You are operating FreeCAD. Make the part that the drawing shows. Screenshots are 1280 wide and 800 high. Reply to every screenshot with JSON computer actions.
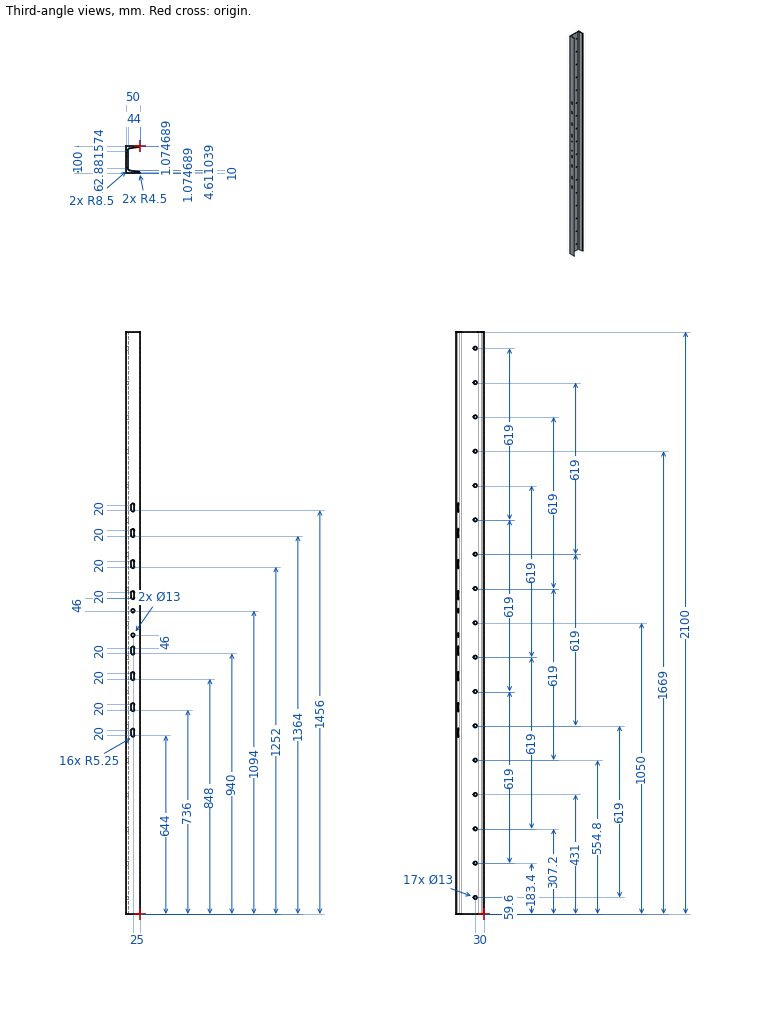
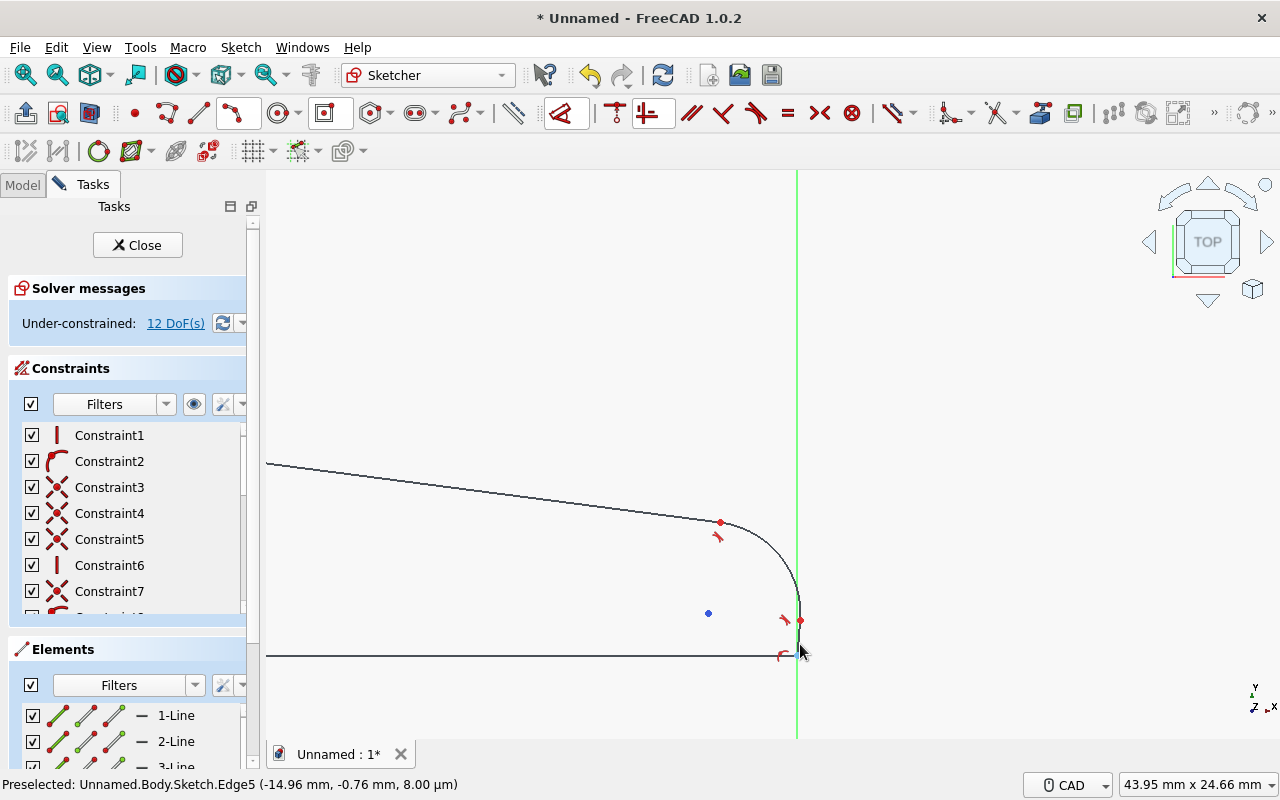
{"action": "left_click", "coordinate": [799, 642]}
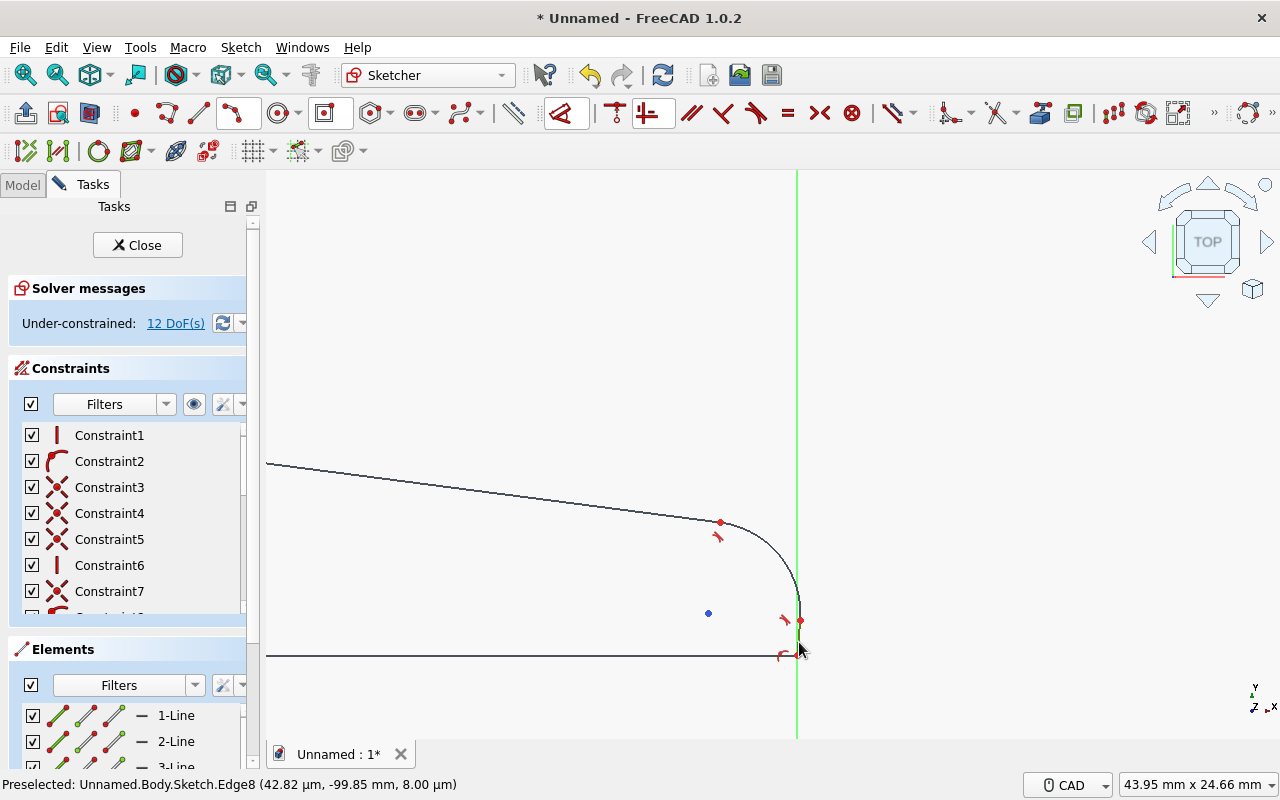
{"action": "left_click", "coordinate": [670, 114]}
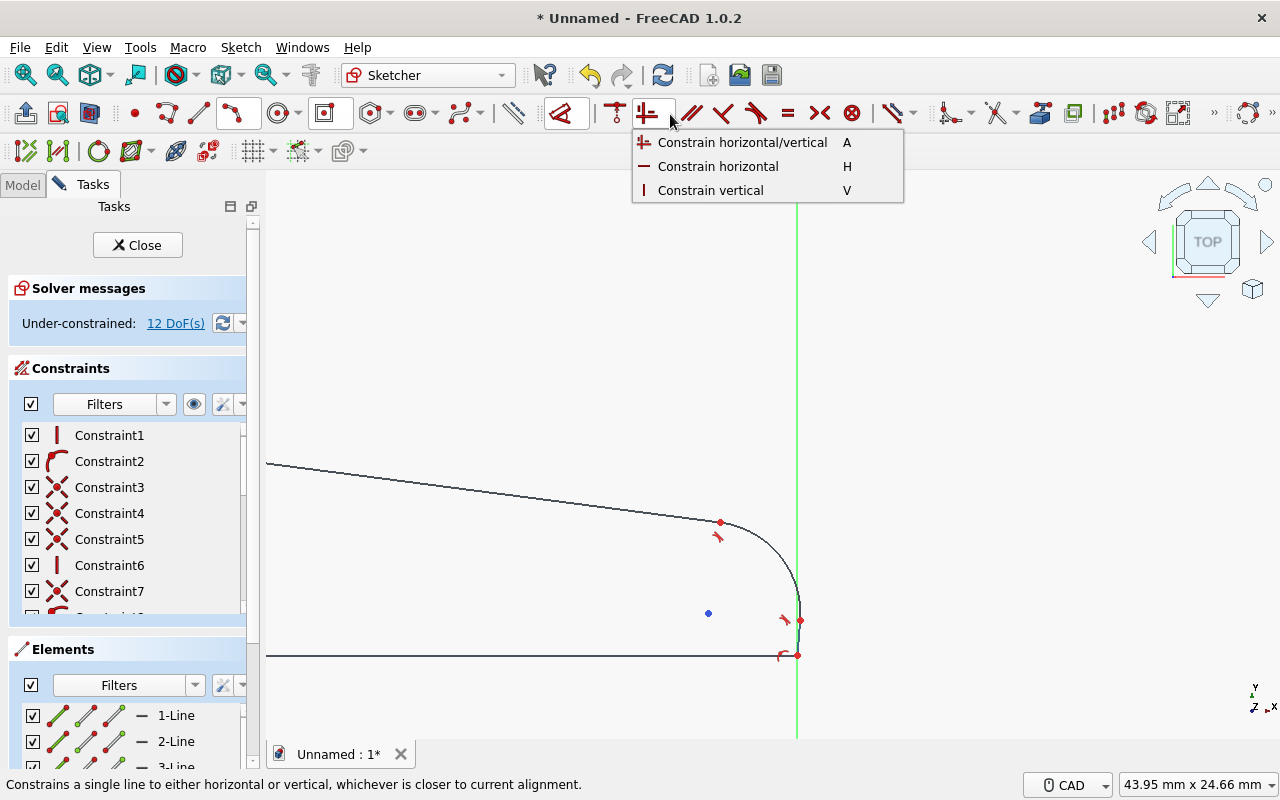
{"action": "left_click", "coordinate": [768, 190]}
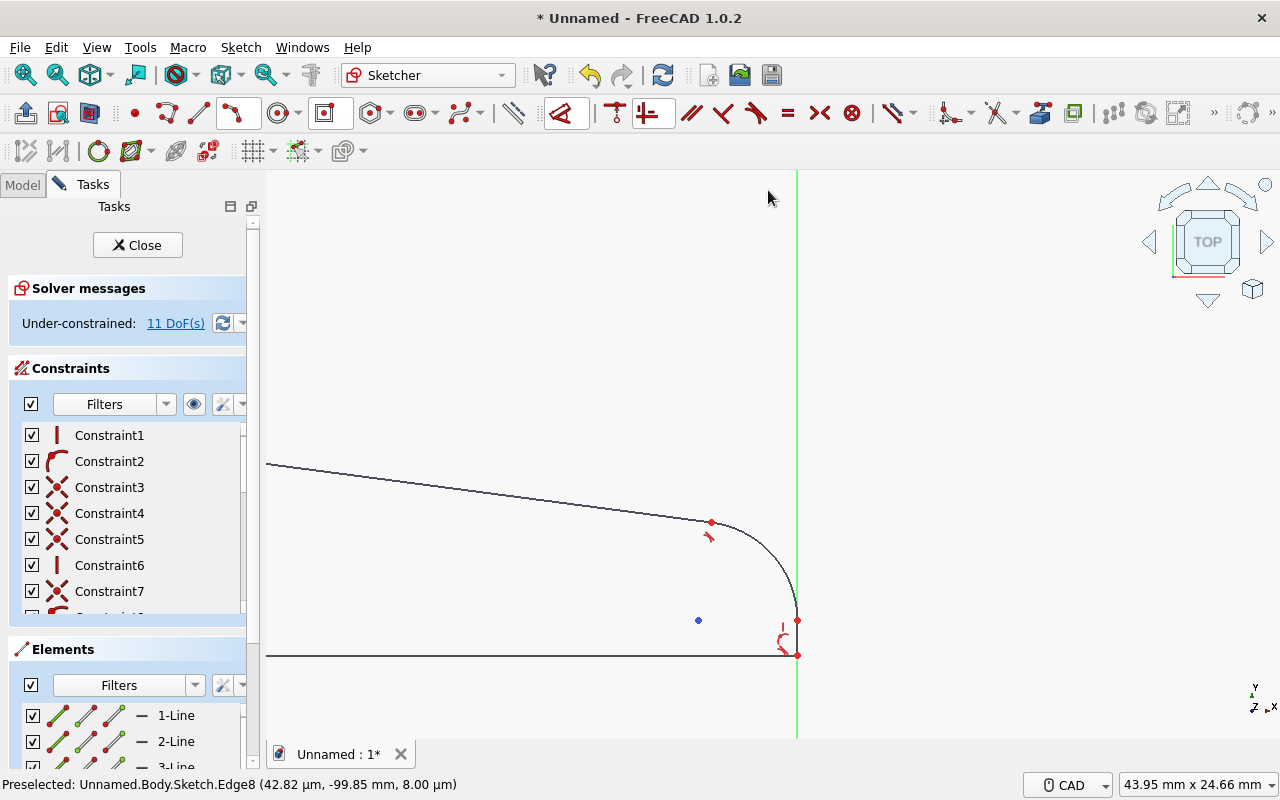
{"action": "scroll", "coordinate": [800, 645], "scroll_direction": "down", "scroll_amount": 9}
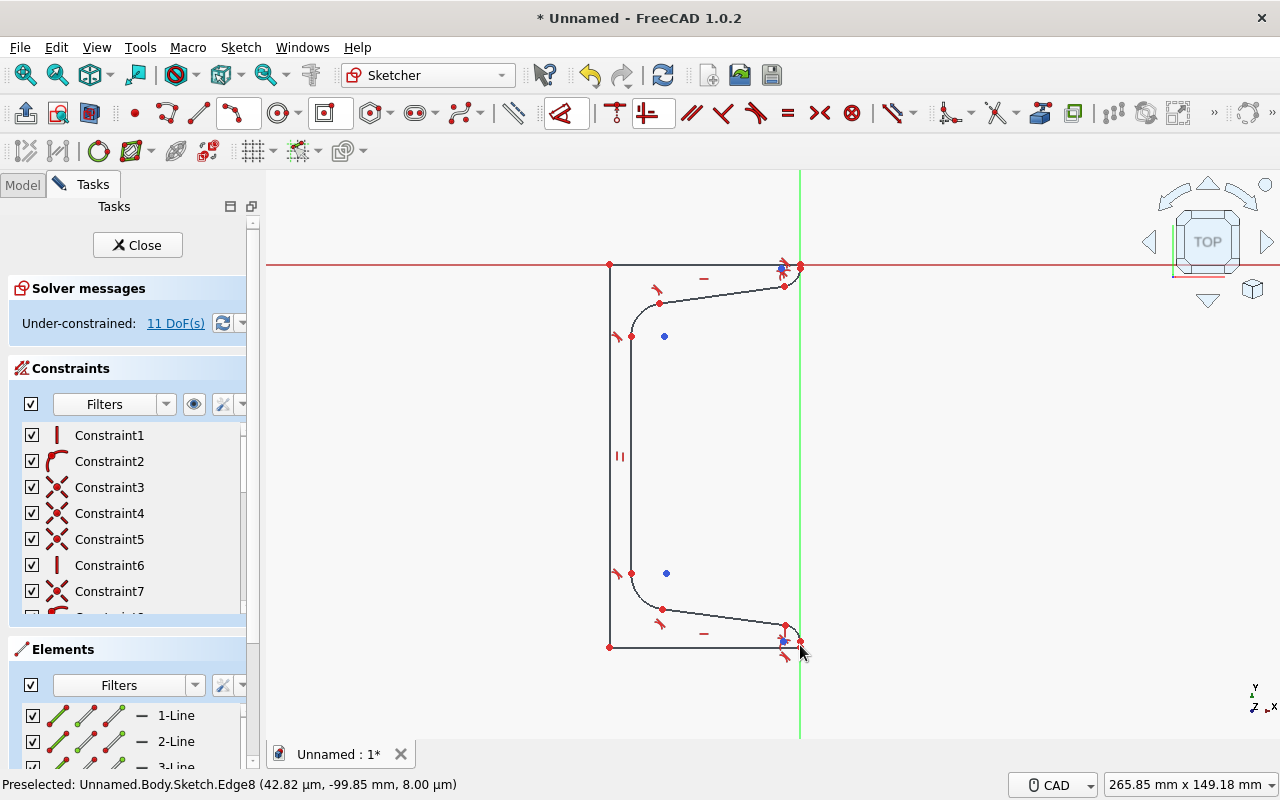
{"action": "left_click", "coordinate": [635, 589]}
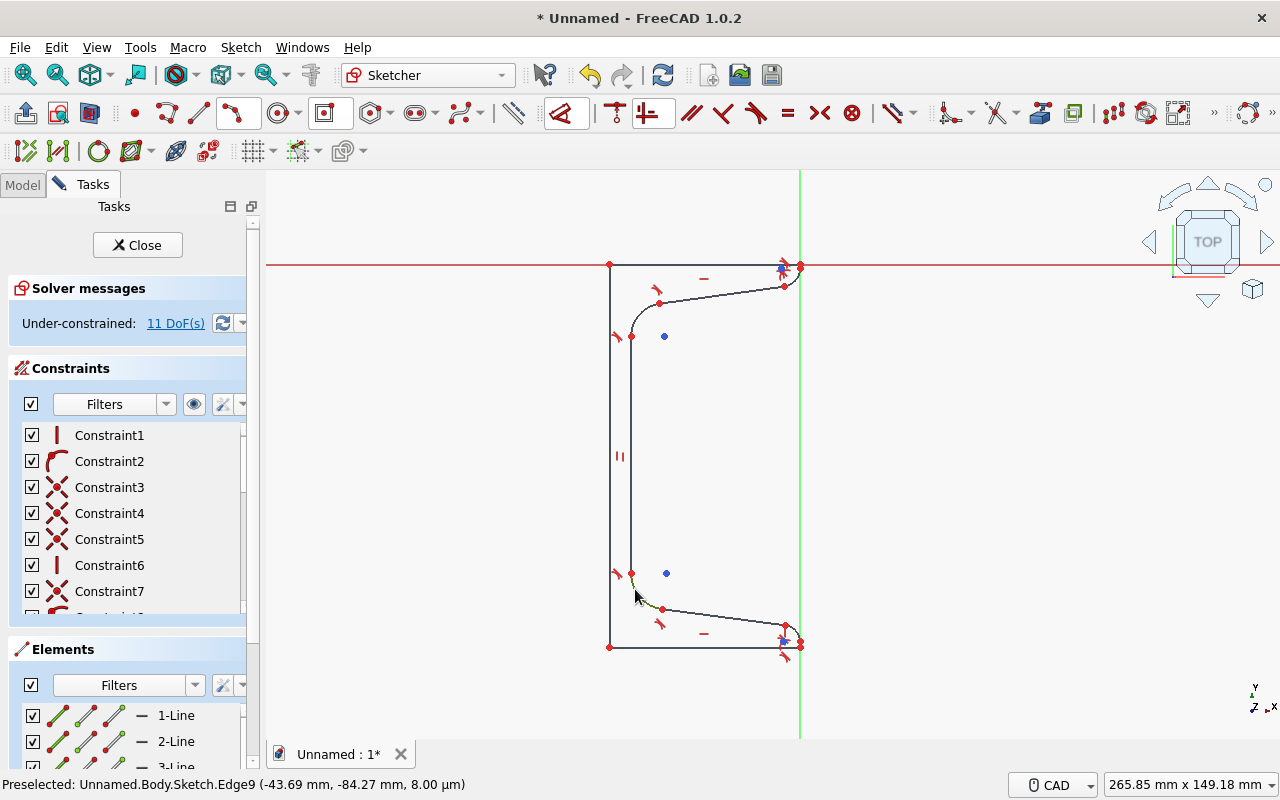
{"action": "left_click", "coordinate": [647, 309]}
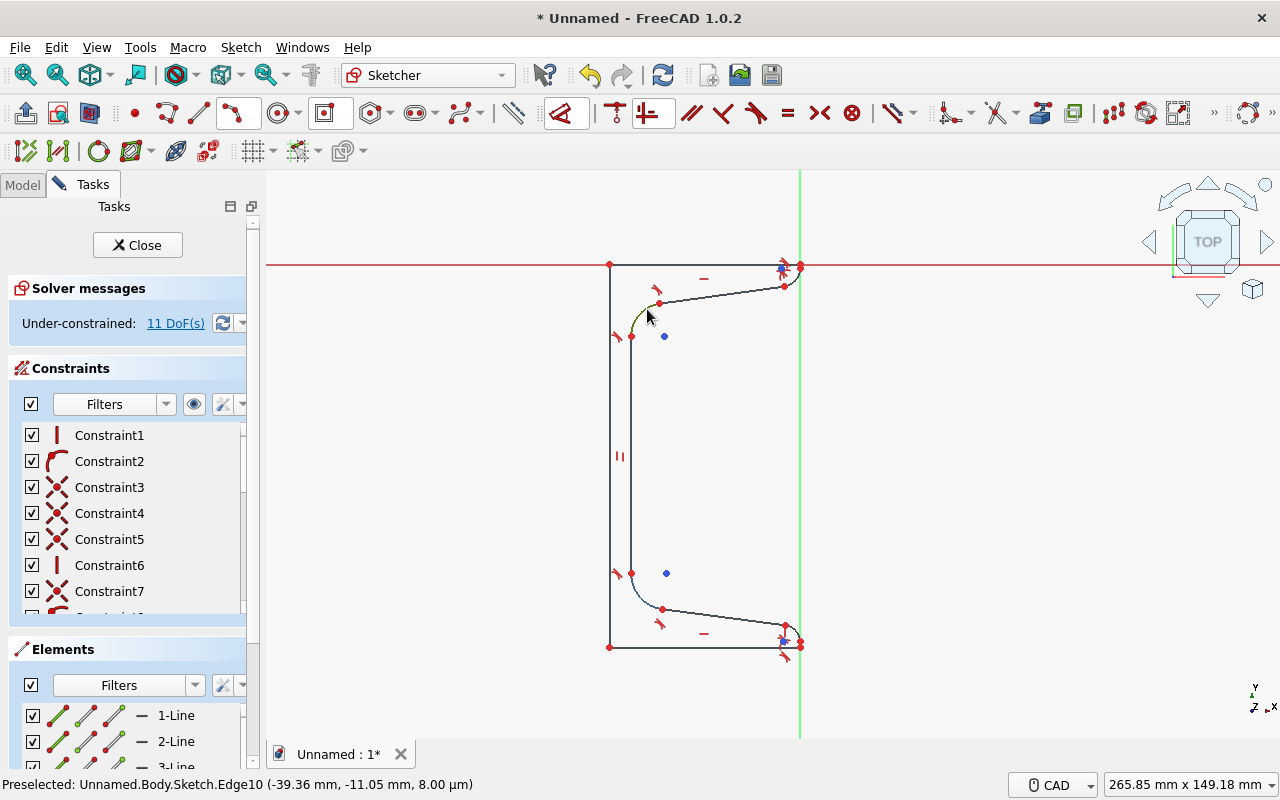
{"action": "key", "text": "e"}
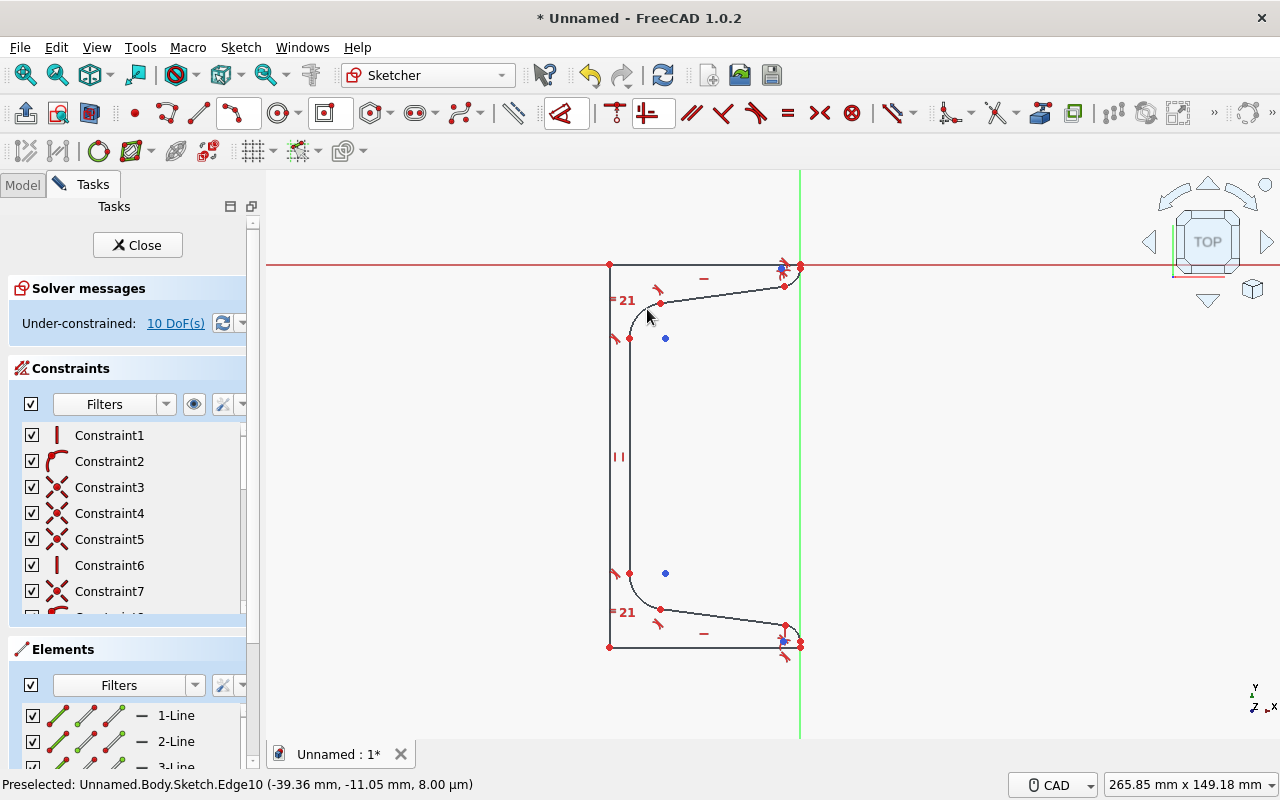
{"action": "scroll", "coordinate": [791, 284], "scroll_direction": "up", "scroll_amount": 3}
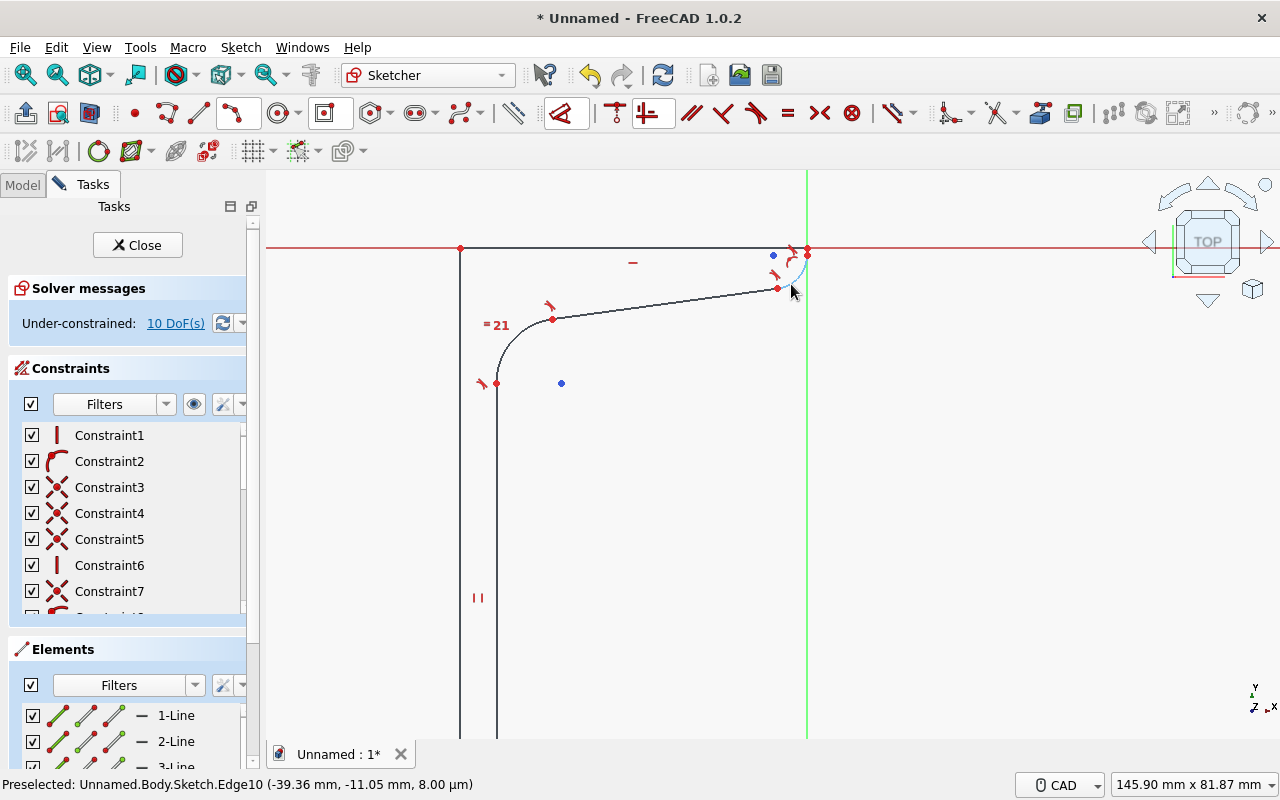
{"action": "left_click", "coordinate": [791, 284]}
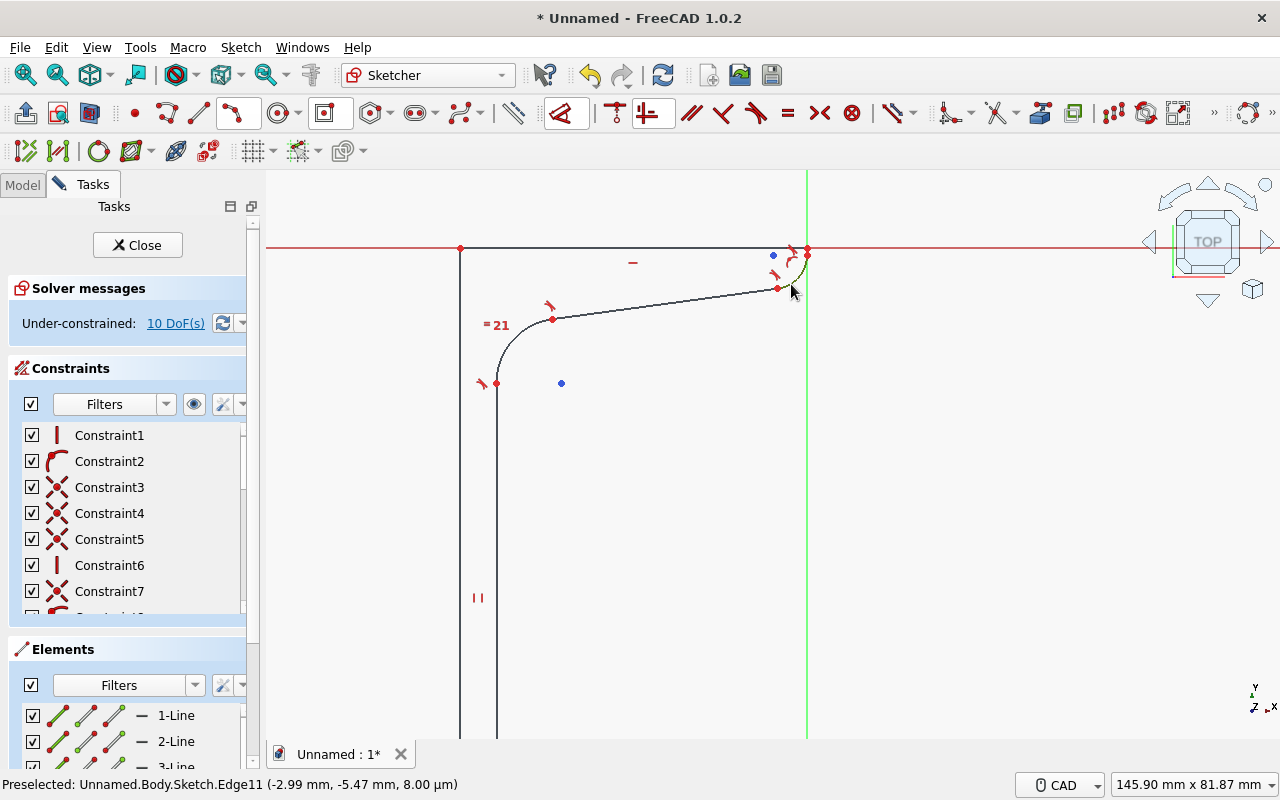
{"action": "scroll", "coordinate": [791, 283], "scroll_direction": "down", "scroll_amount": 3}